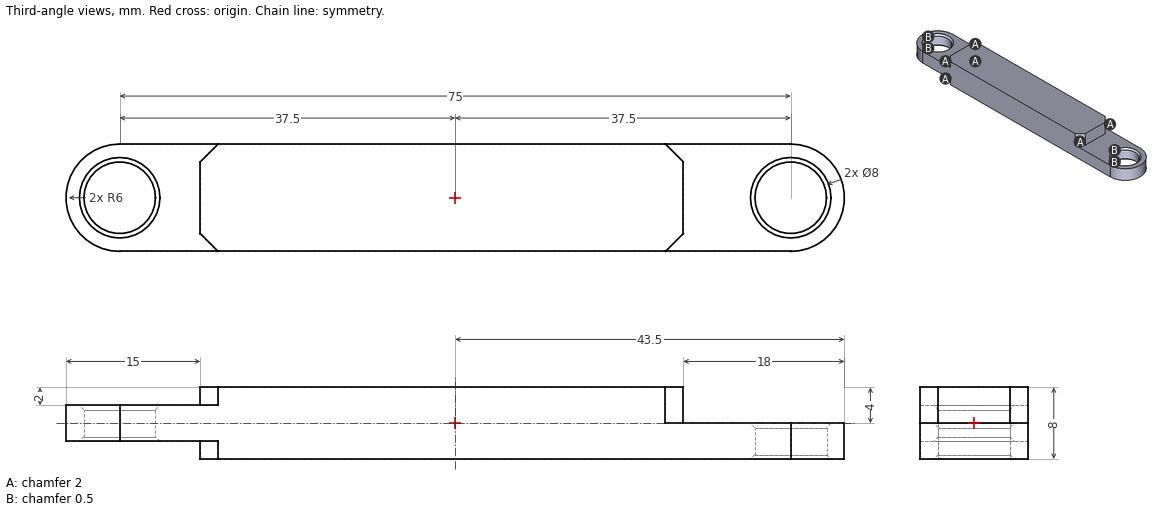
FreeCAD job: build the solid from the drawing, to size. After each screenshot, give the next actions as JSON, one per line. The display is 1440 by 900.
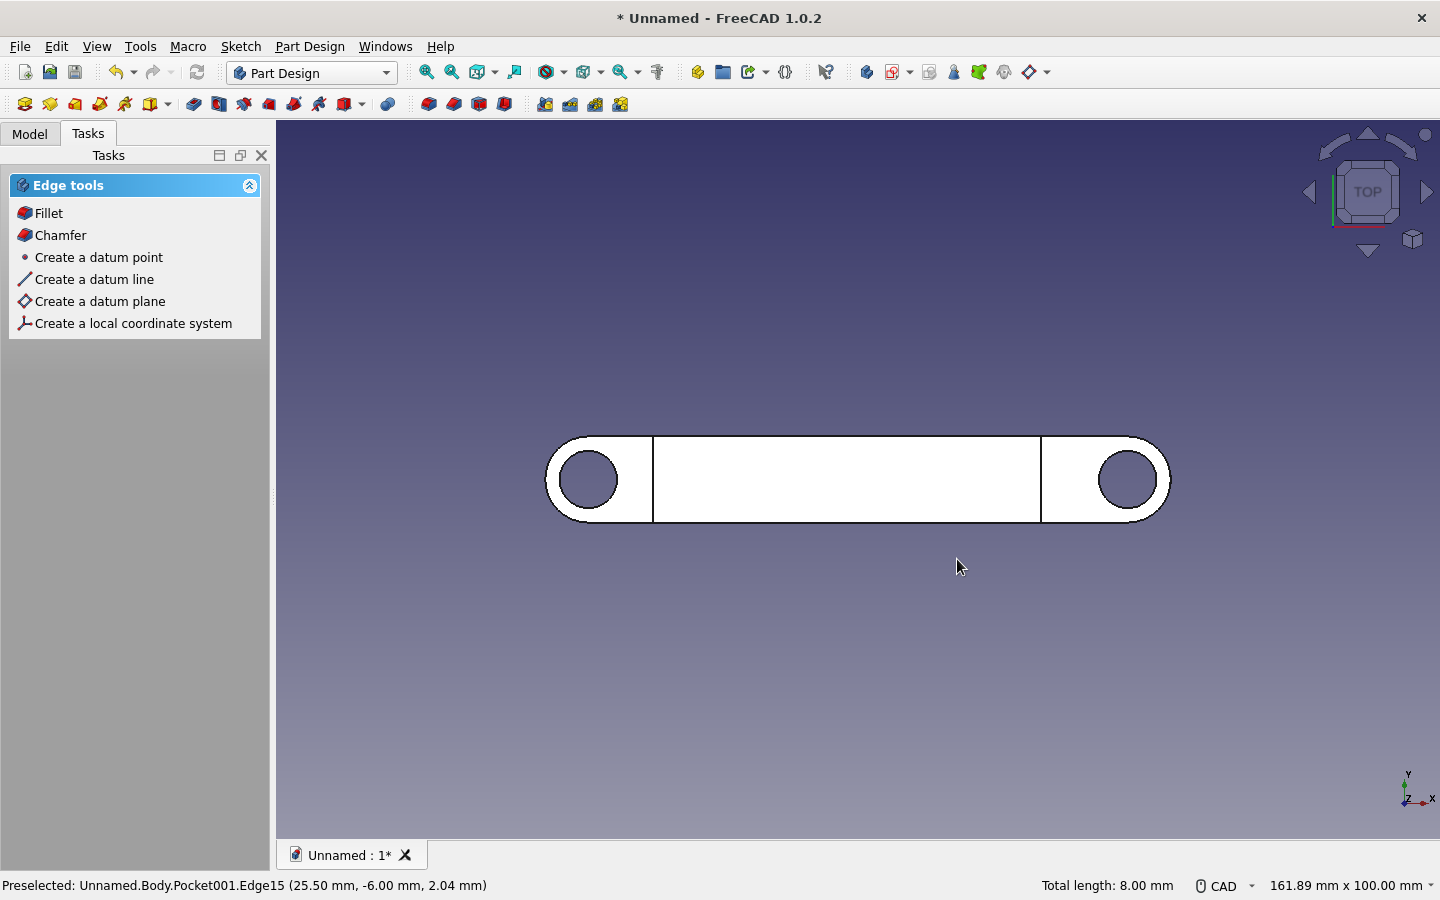
{"action": "key", "text": "1"}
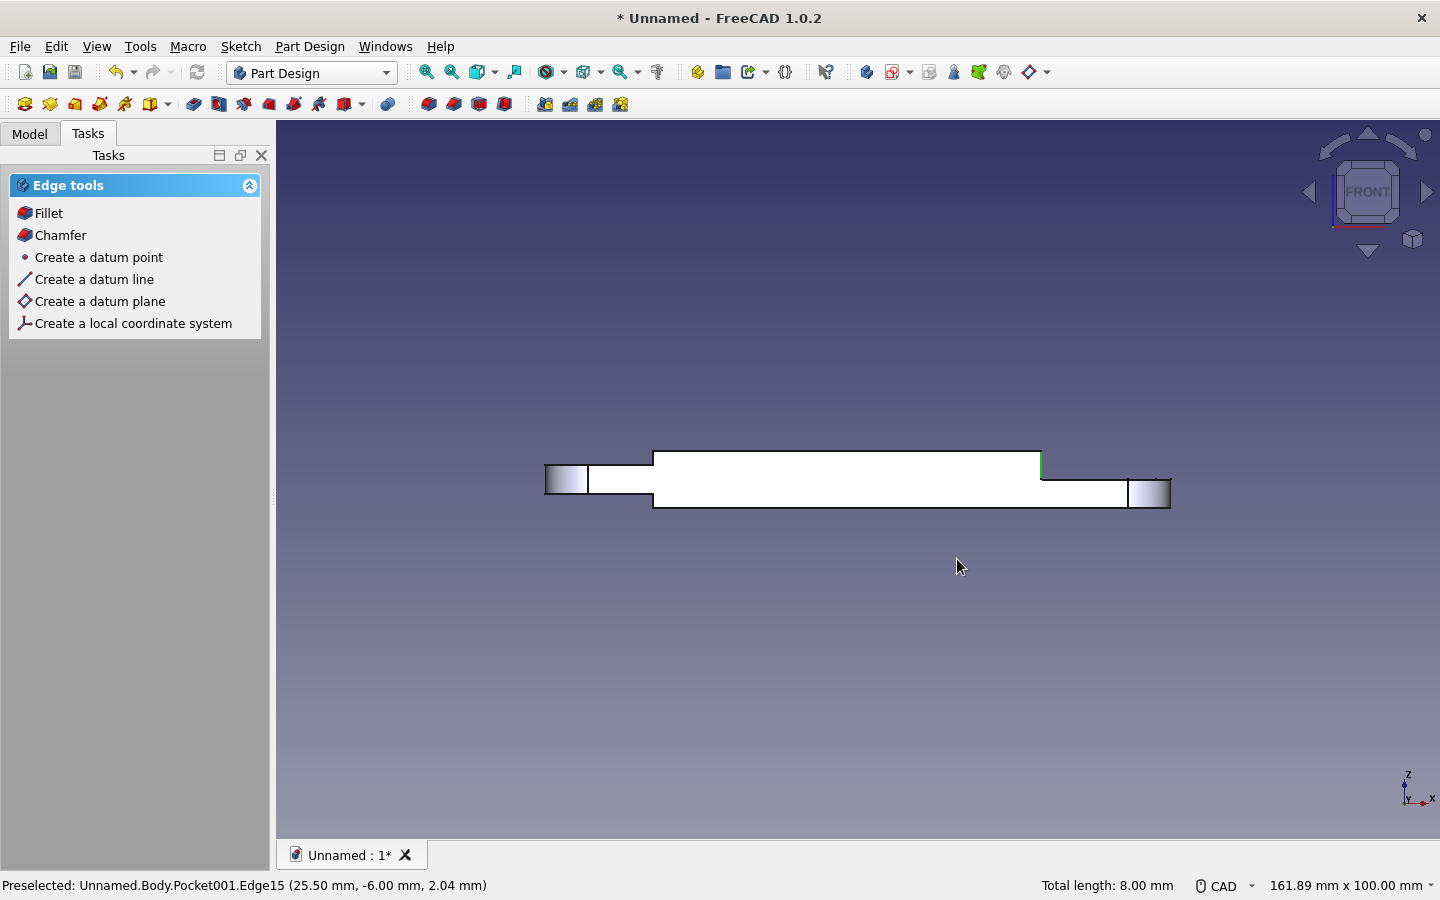
{"action": "left_click", "coordinate": [653, 457], "text": "ctrl"}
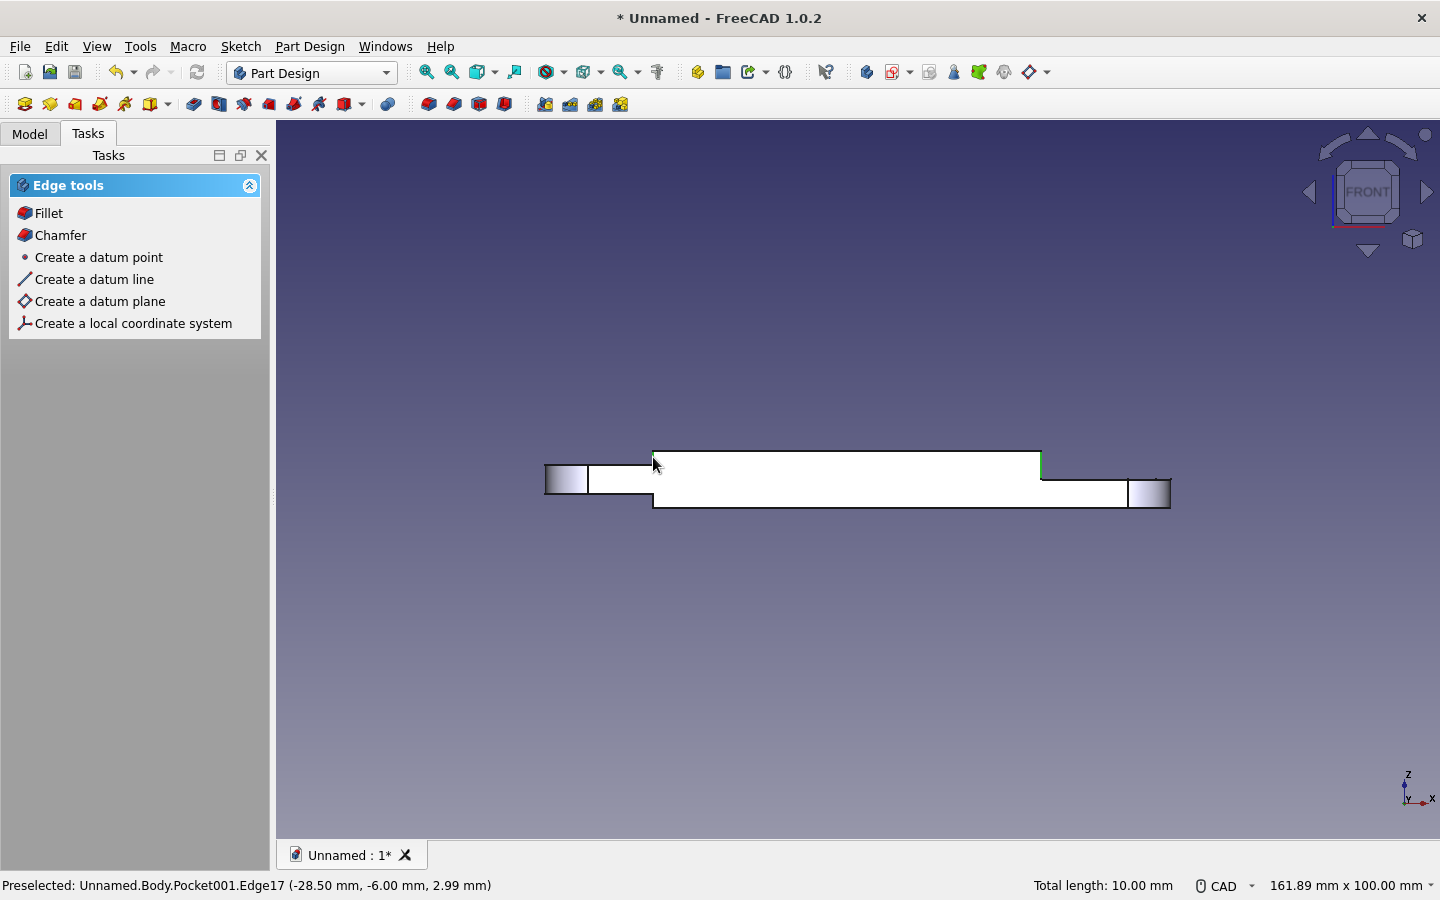
{"action": "left_click", "coordinate": [653, 500], "text": "ctrl"}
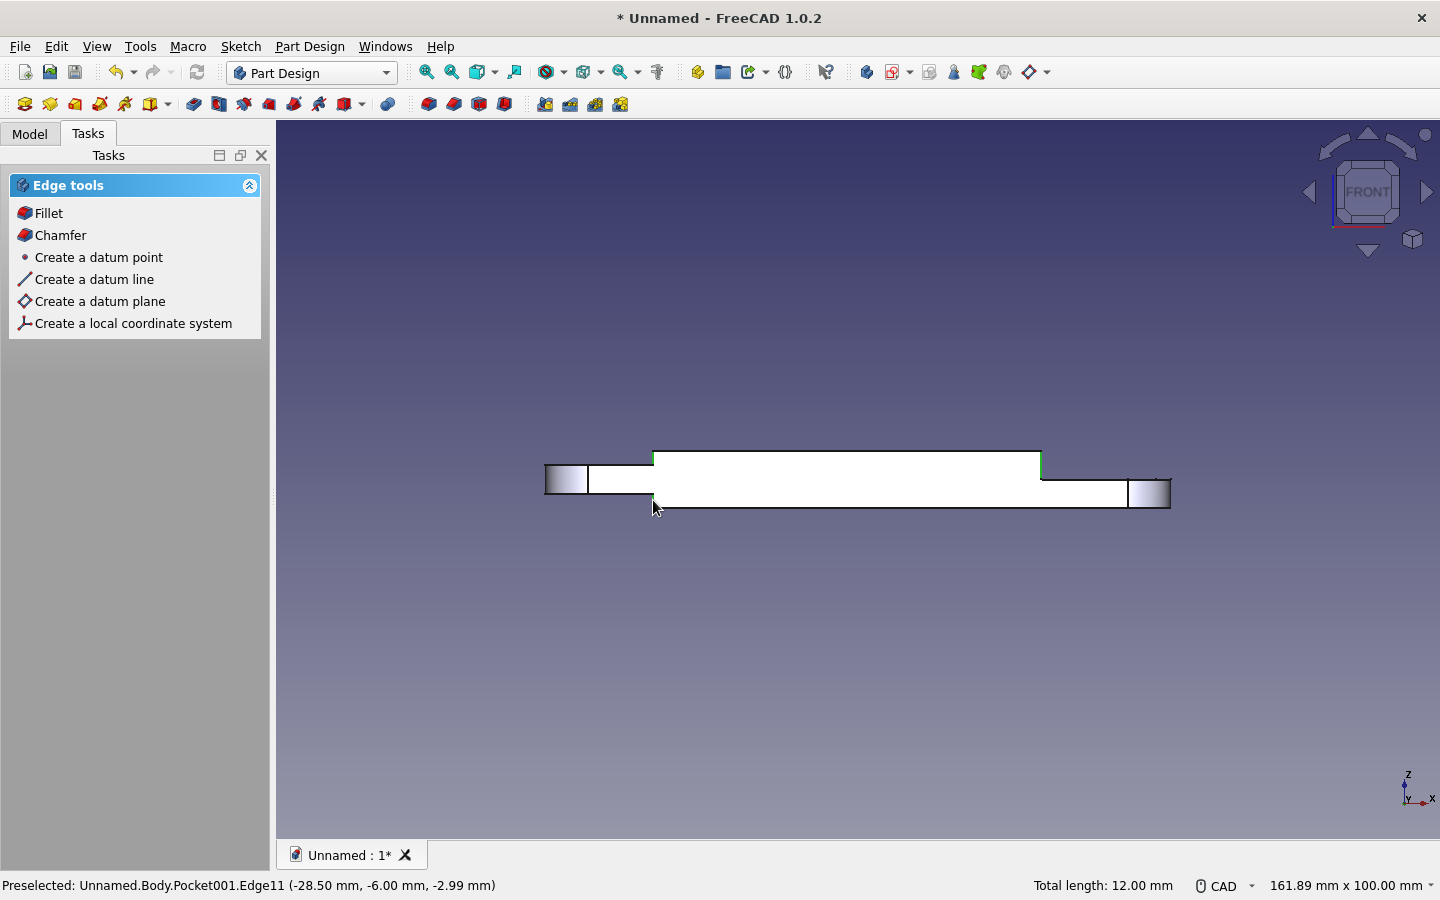
{"action": "key", "text": "3"}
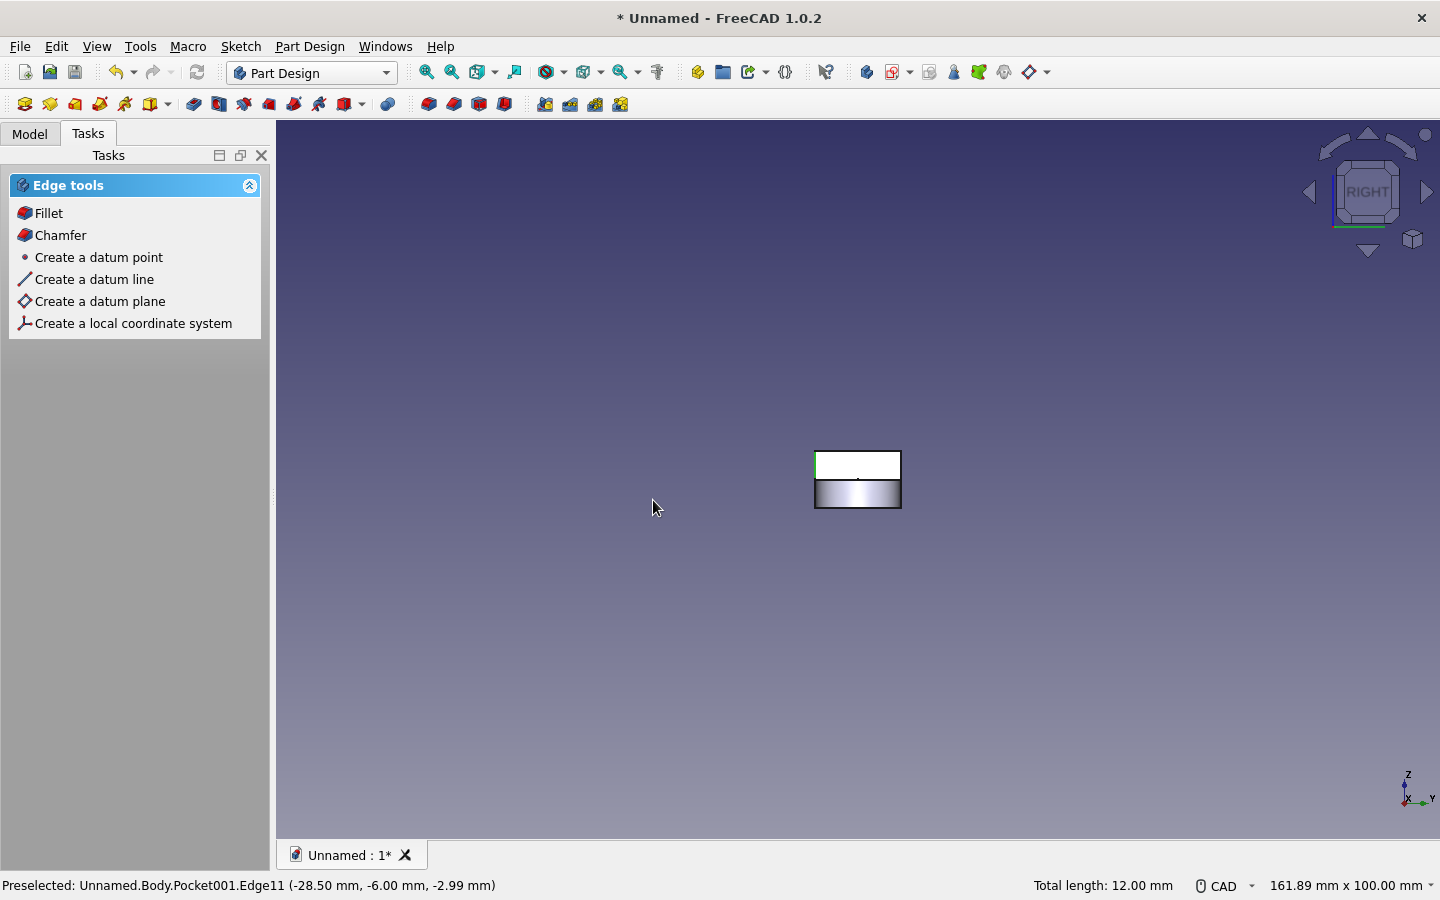
{"action": "left_click", "coordinate": [427, 72]}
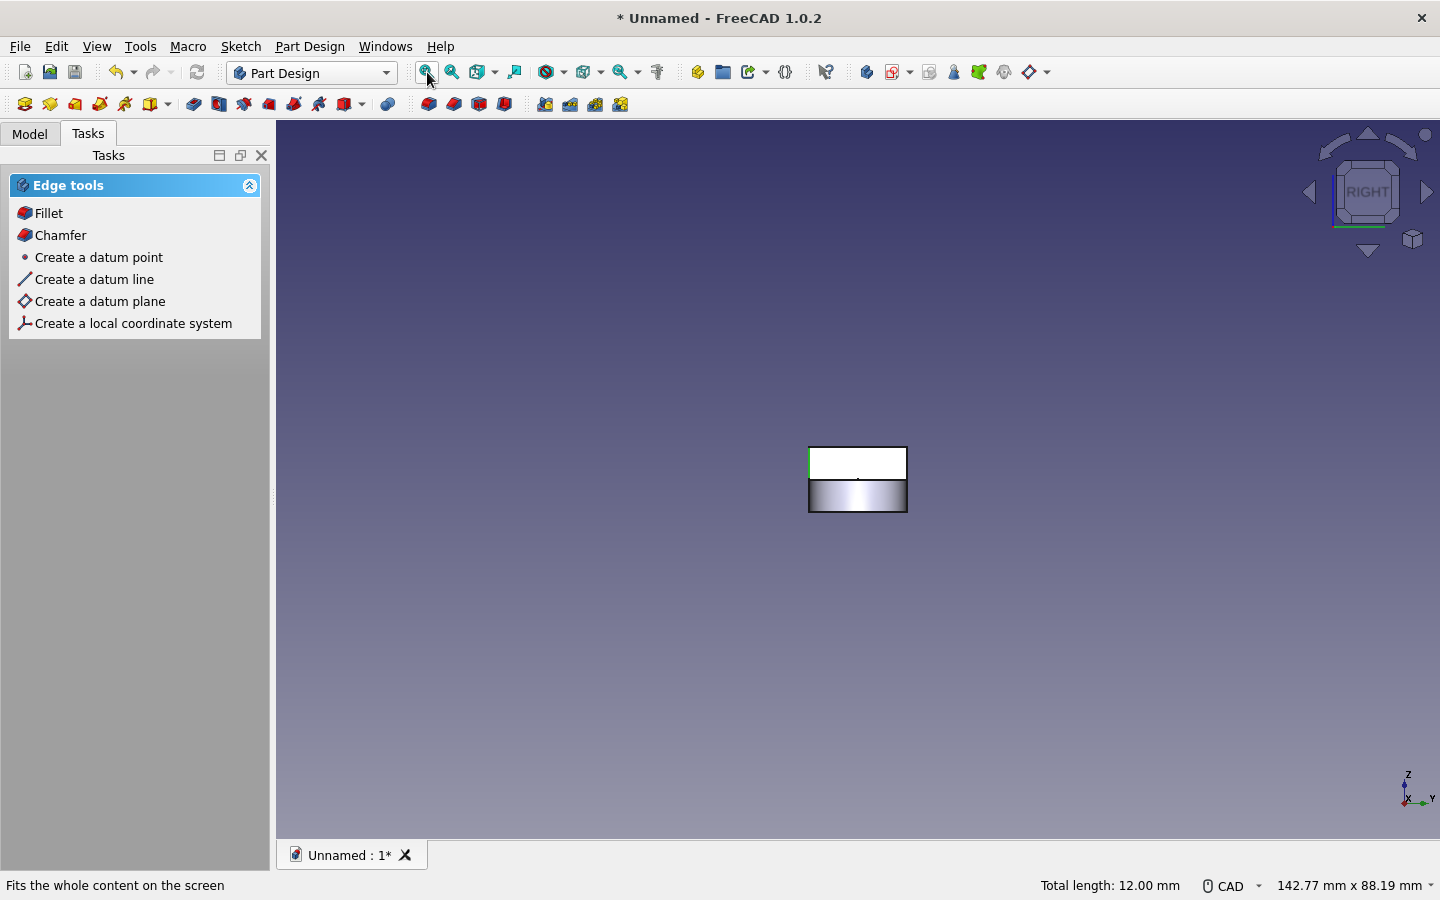
{"action": "left_click", "coordinate": [907, 462], "text": "ctrl"}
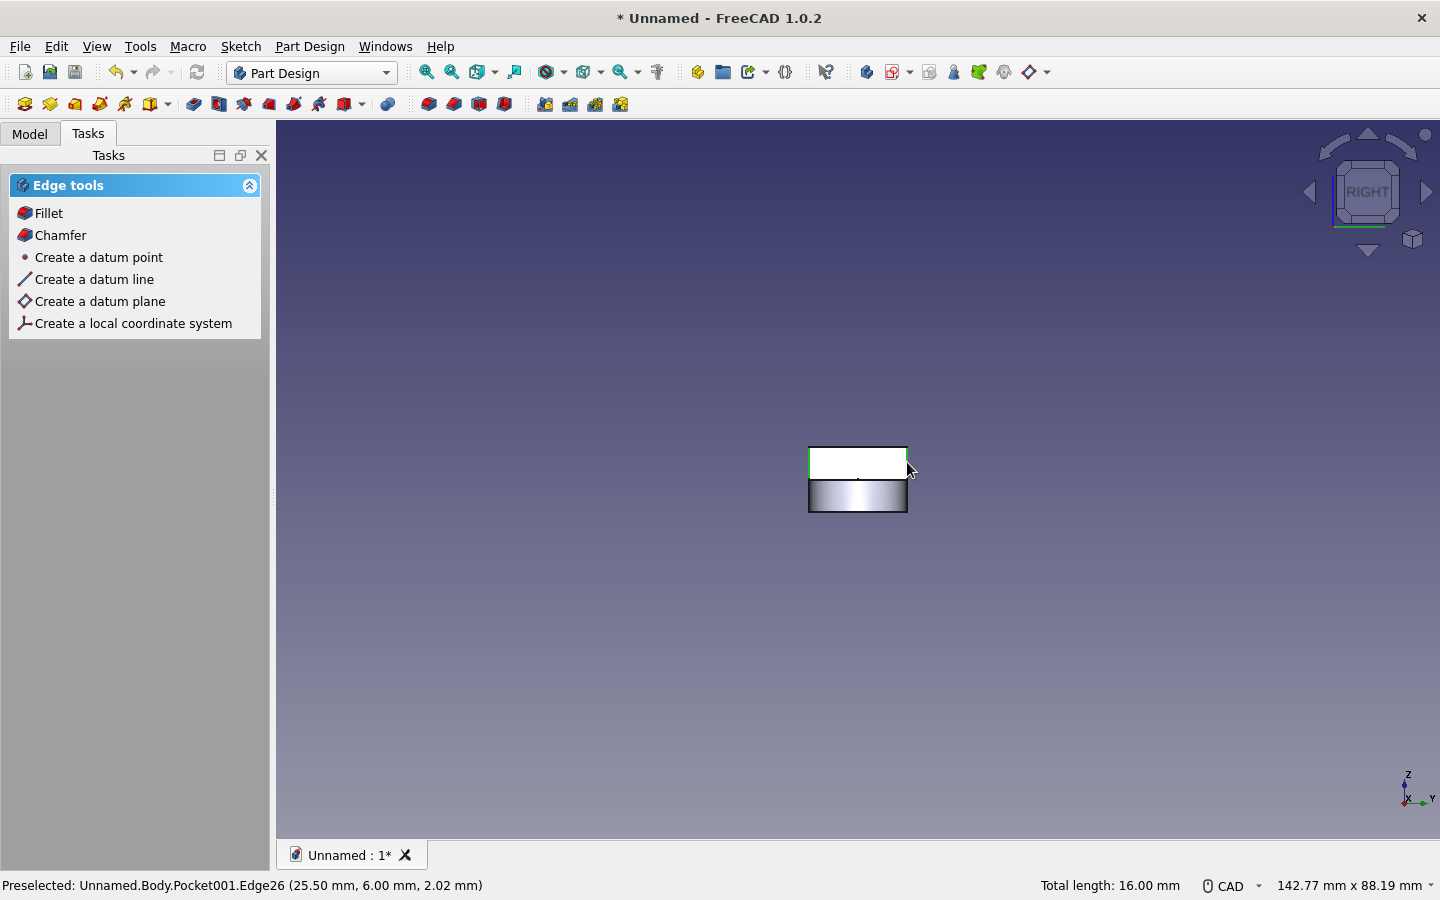
{"action": "left_click", "coordinate": [454, 104]}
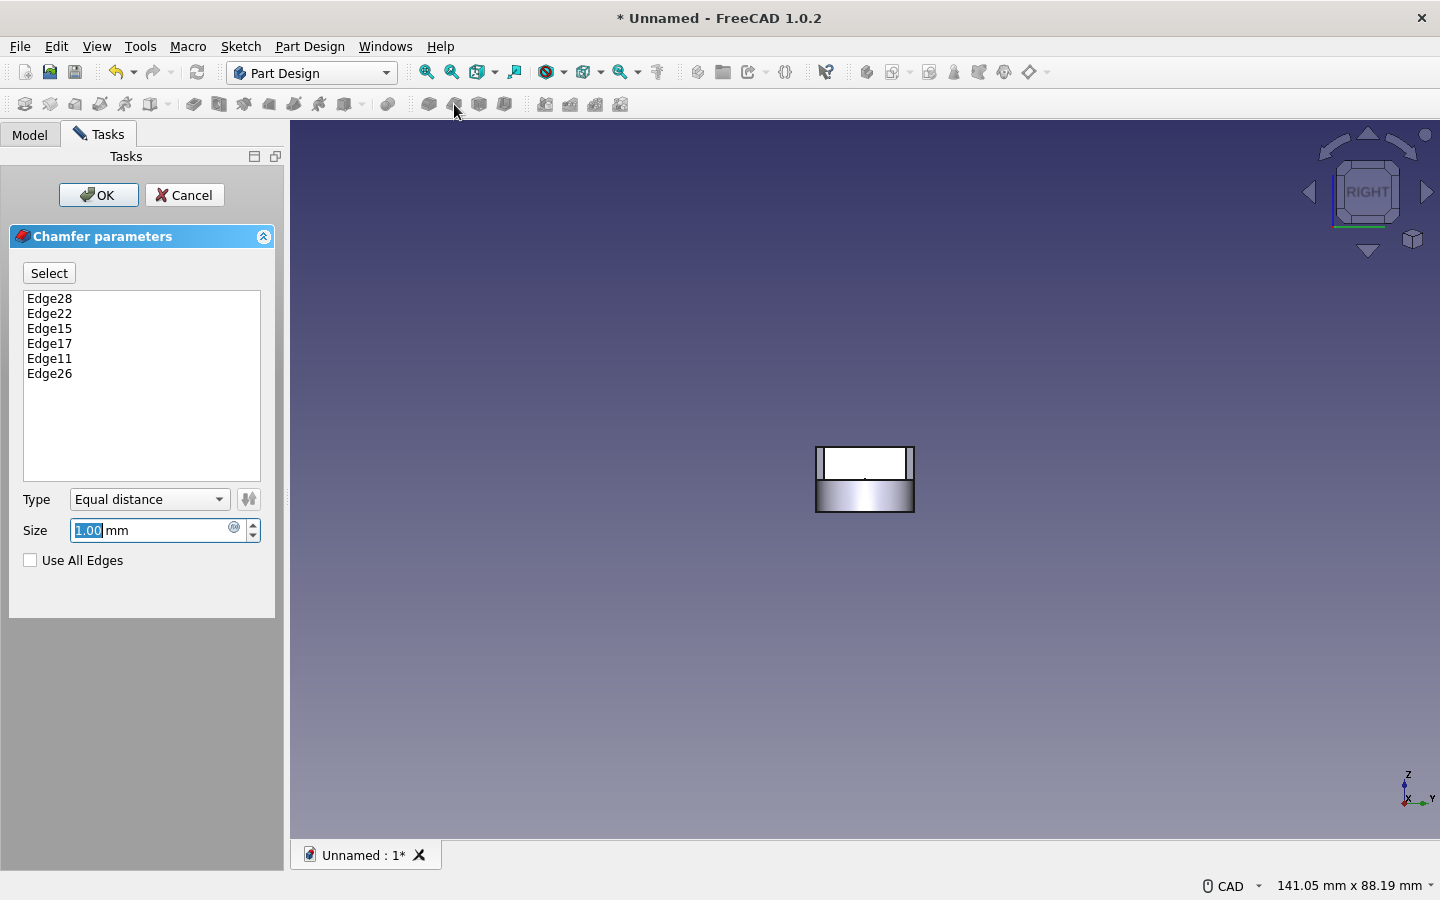
{"action": "type", "text": "2"}
{"action": "key", "text": "Tab"}